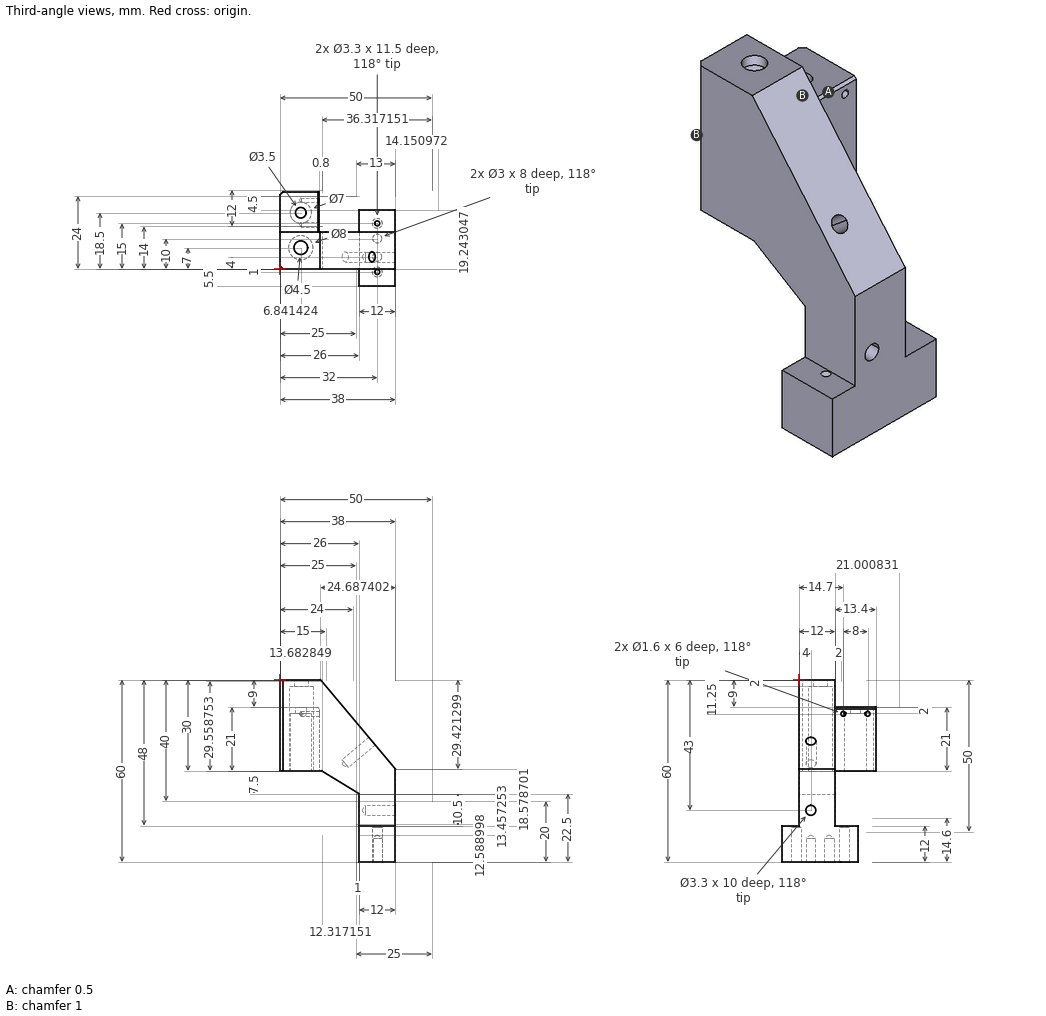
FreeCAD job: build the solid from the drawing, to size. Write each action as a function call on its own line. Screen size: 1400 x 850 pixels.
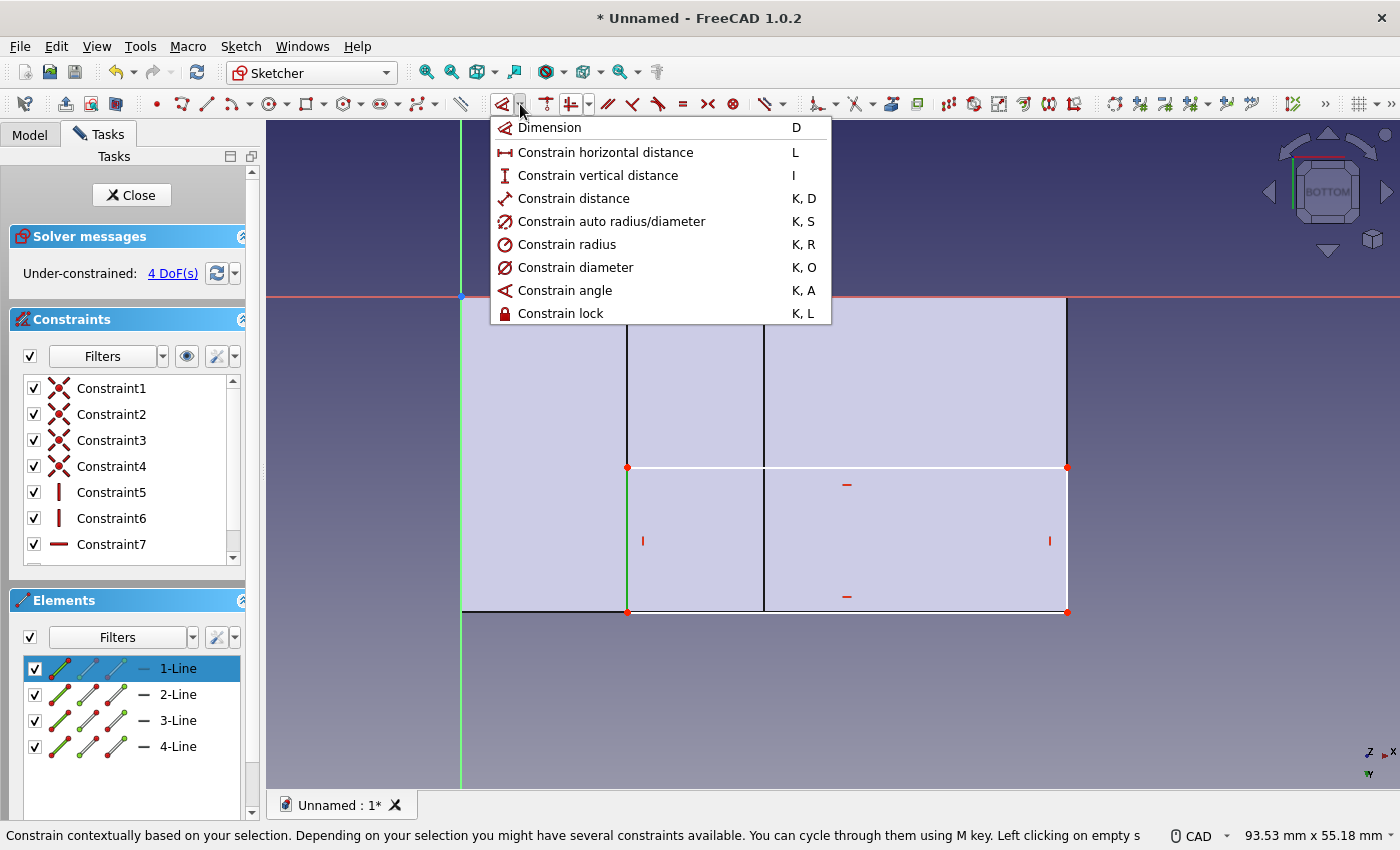
click(661, 176)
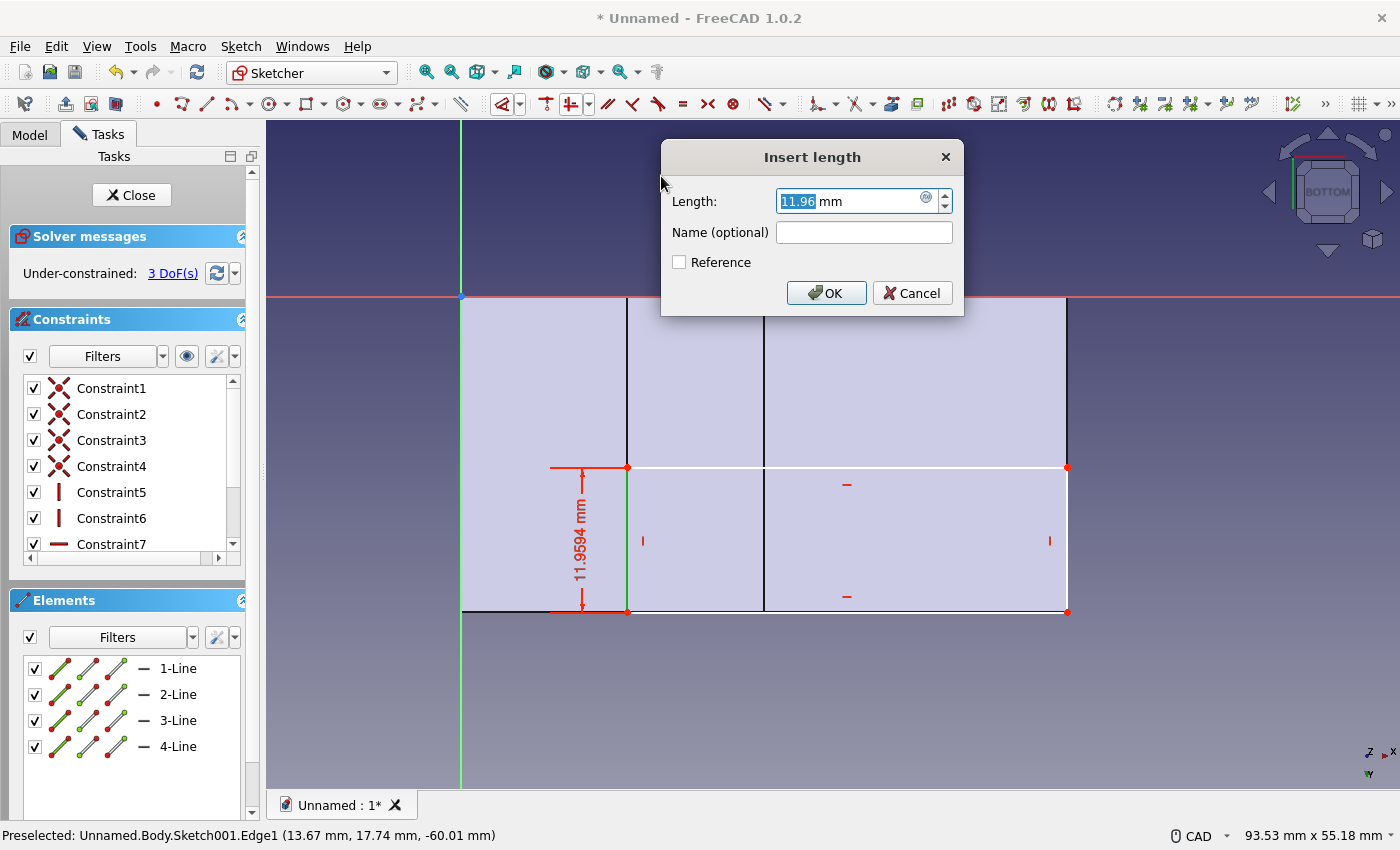
text(12)
key(Return)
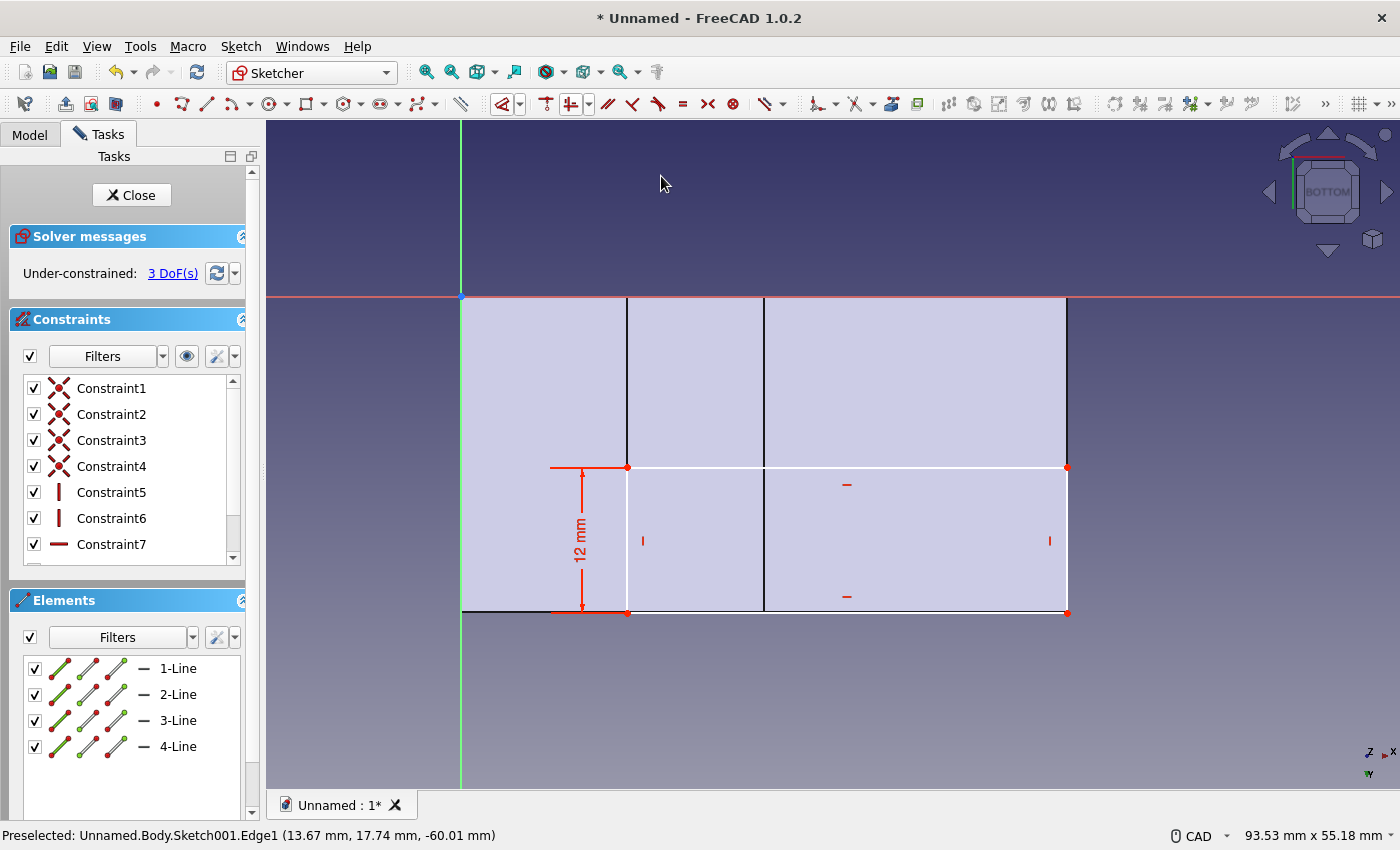
click(627, 468)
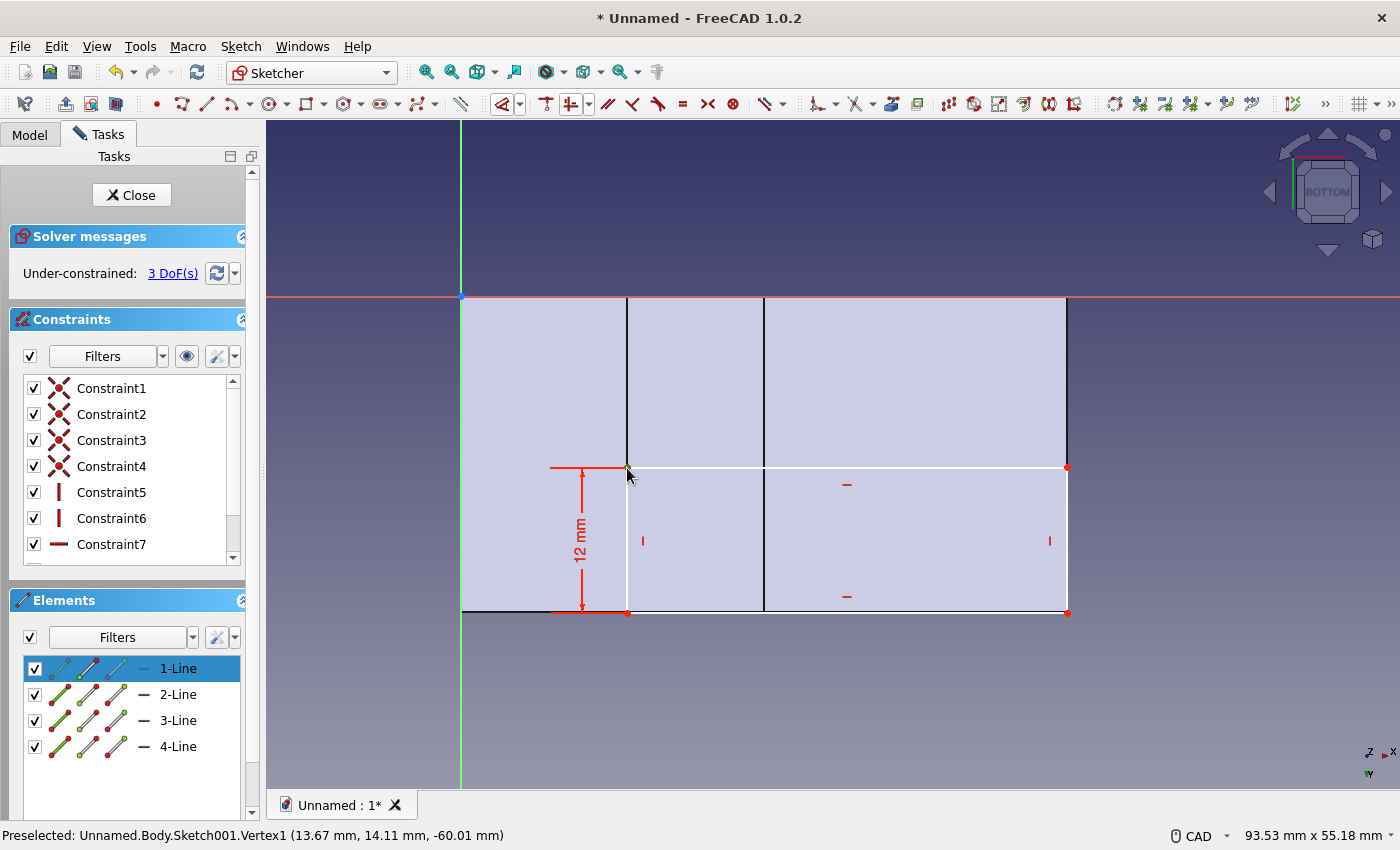
key(i)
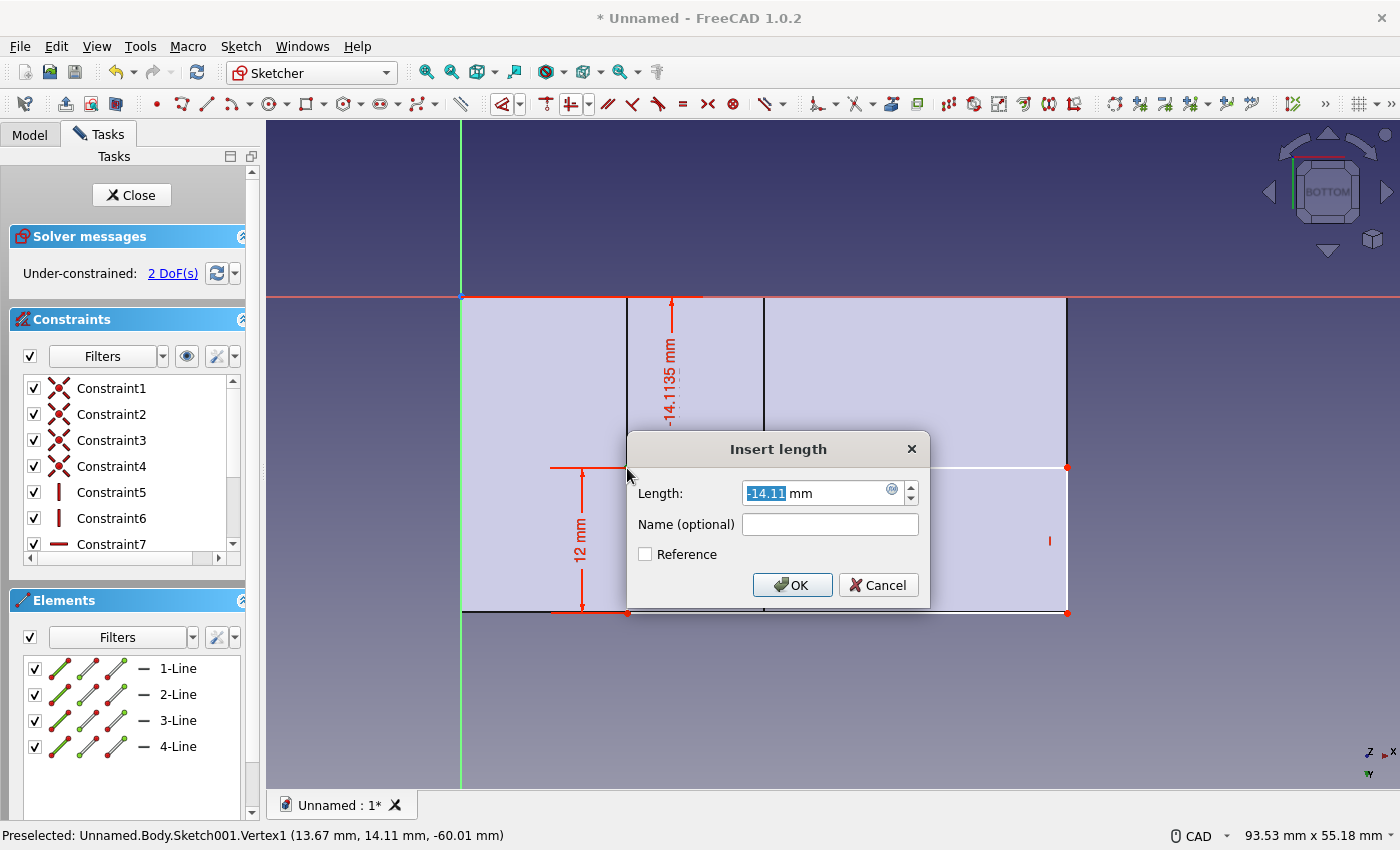
text(-14)
key(Return)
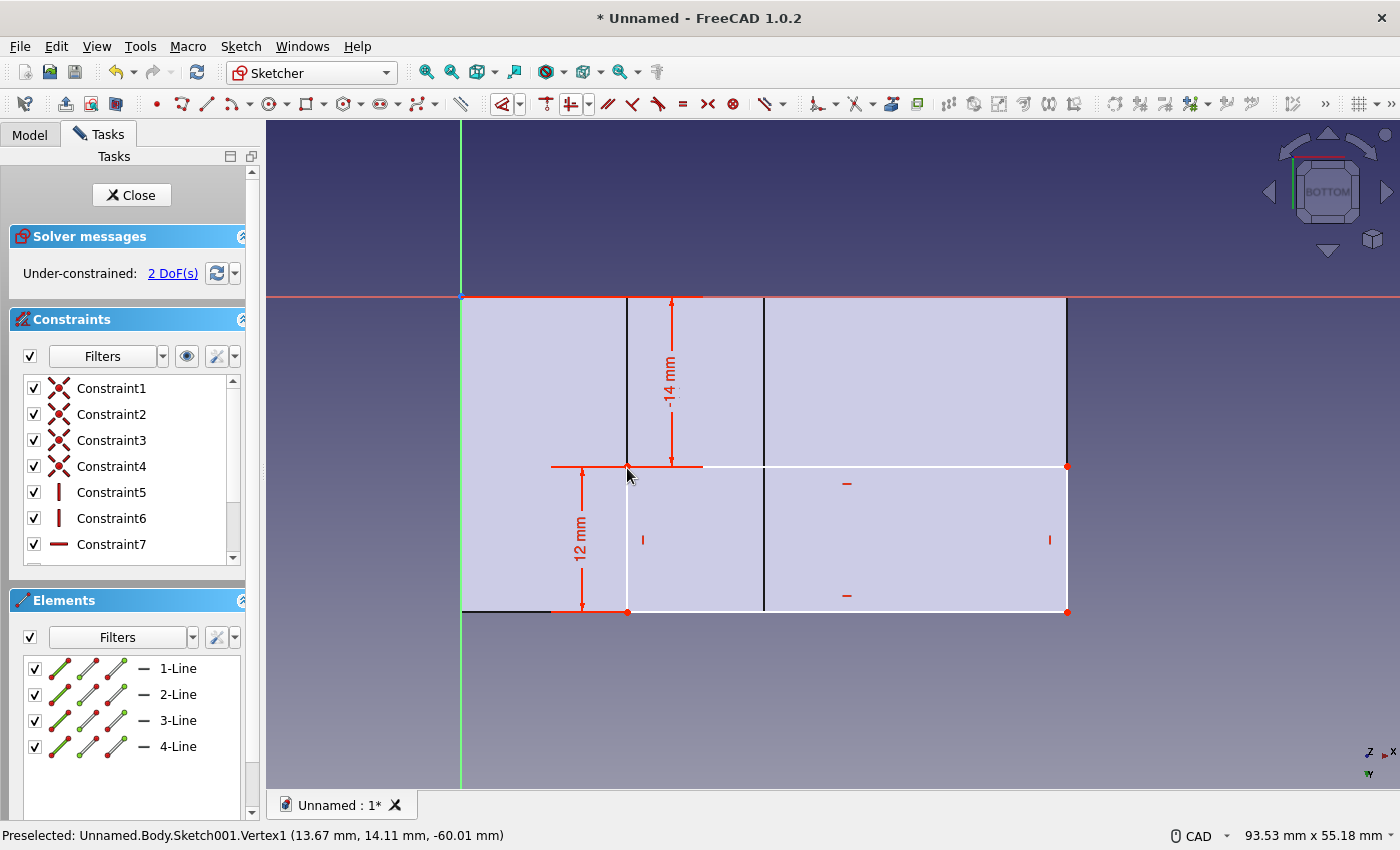
click(1067, 612)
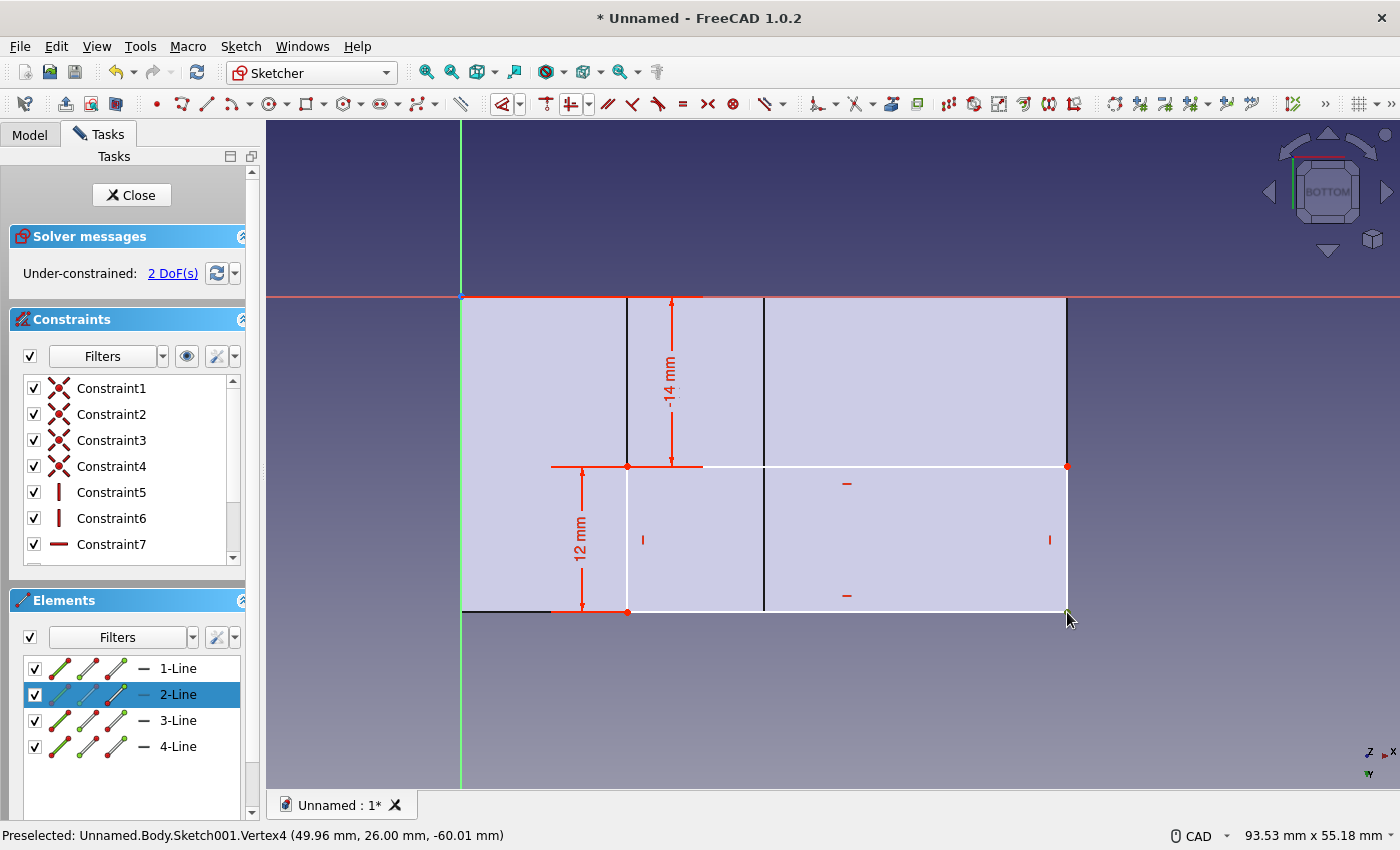
key(l)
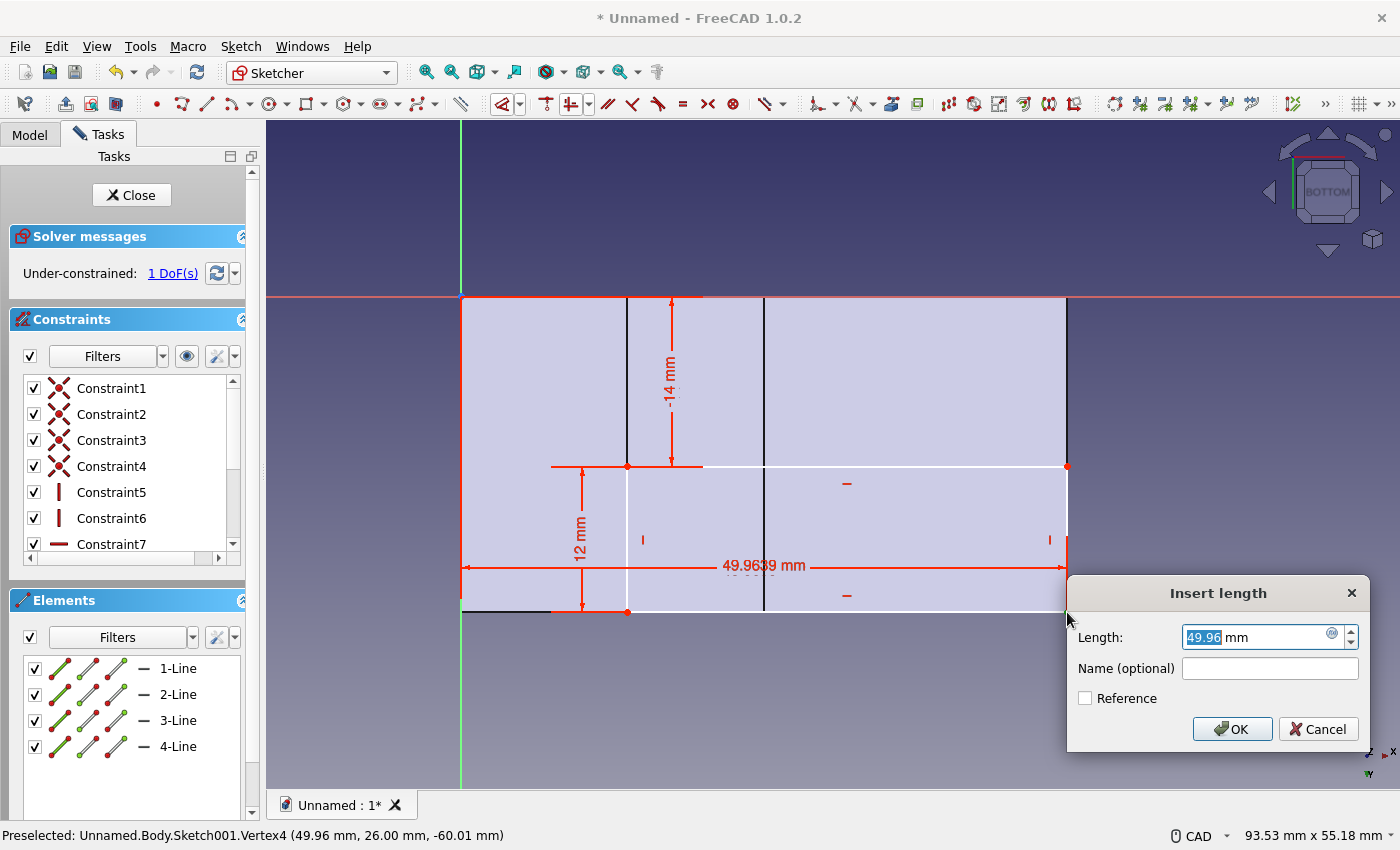
text(50)
key(Return)